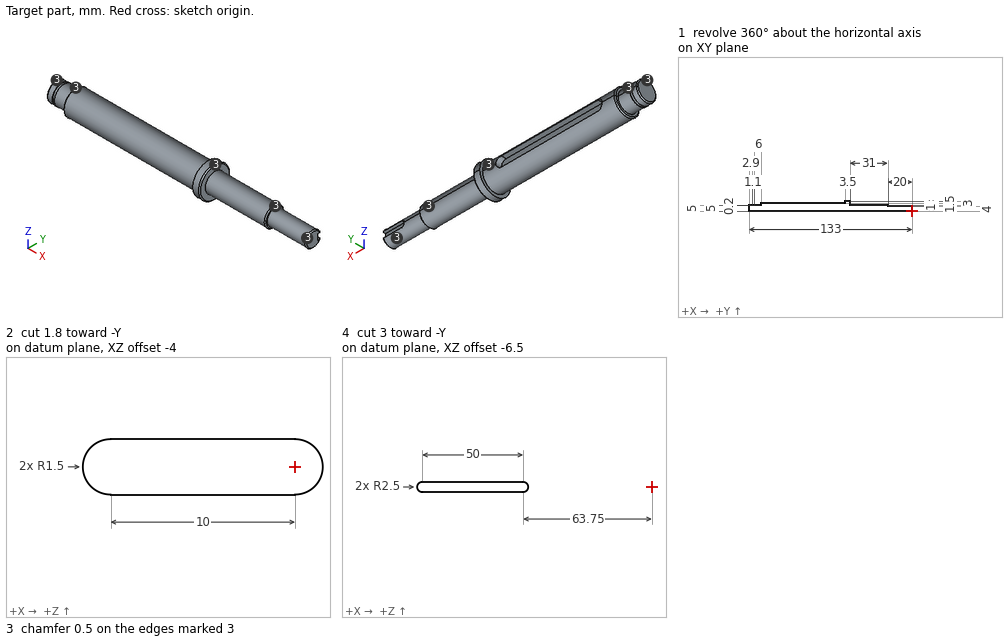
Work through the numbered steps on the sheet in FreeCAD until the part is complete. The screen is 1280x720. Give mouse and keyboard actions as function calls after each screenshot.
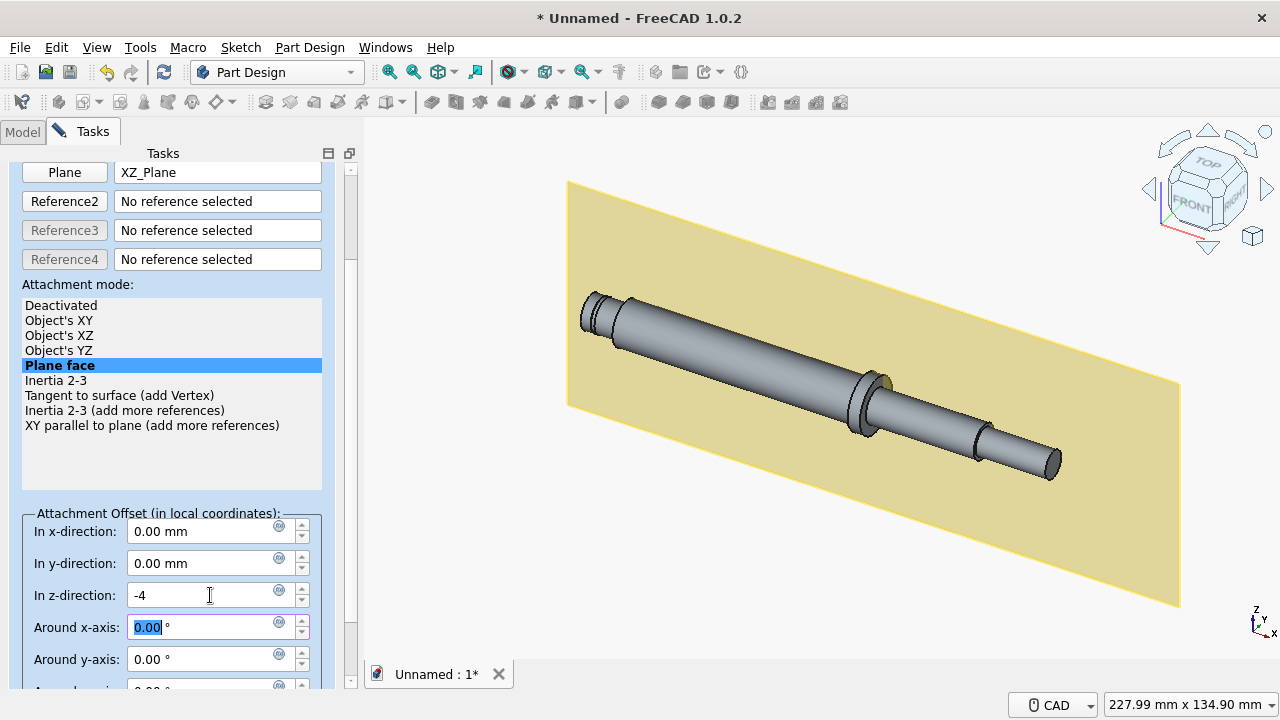
scroll(351, 426, up, 3)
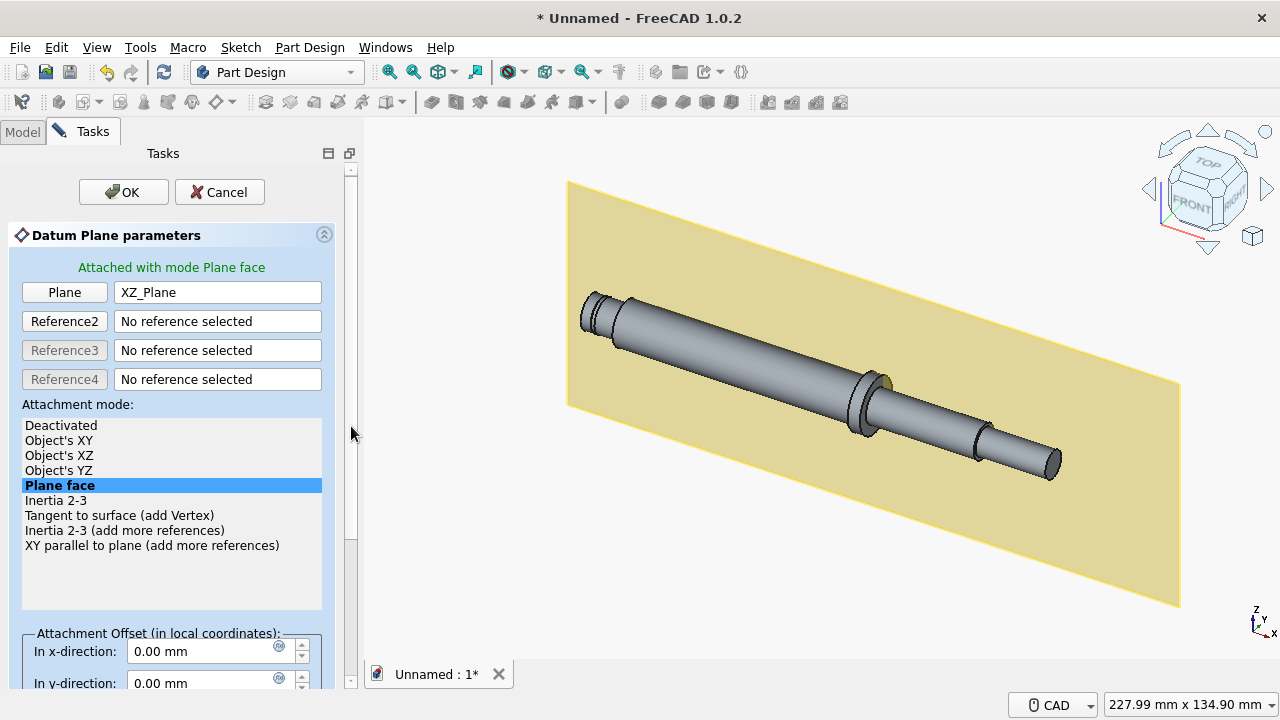
click(124, 192)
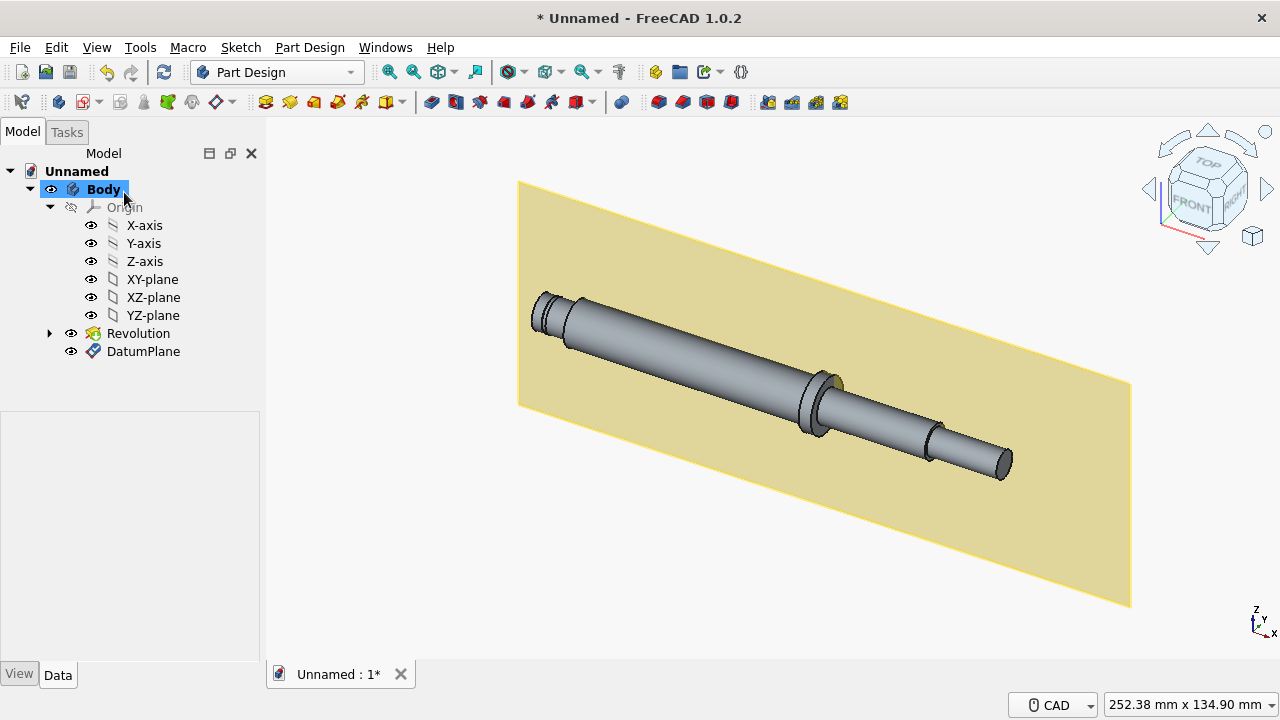
click(116, 351)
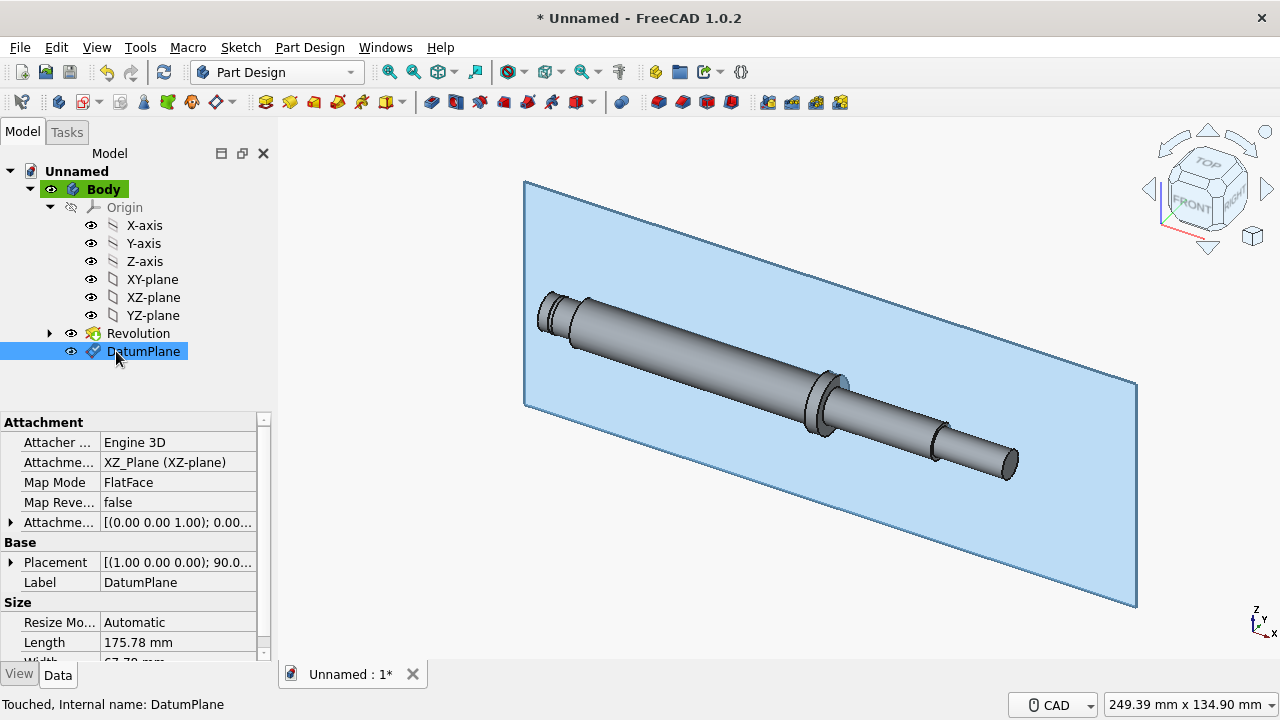
click(84, 102)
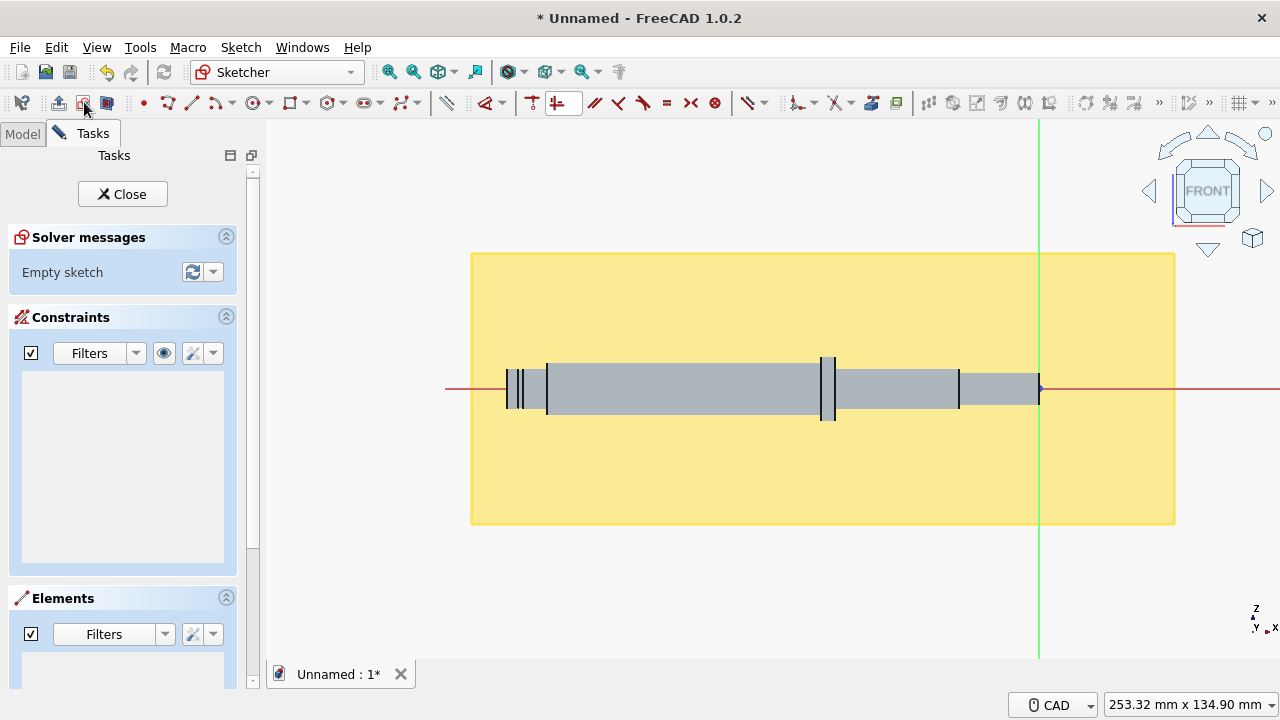
key(q)
key(s)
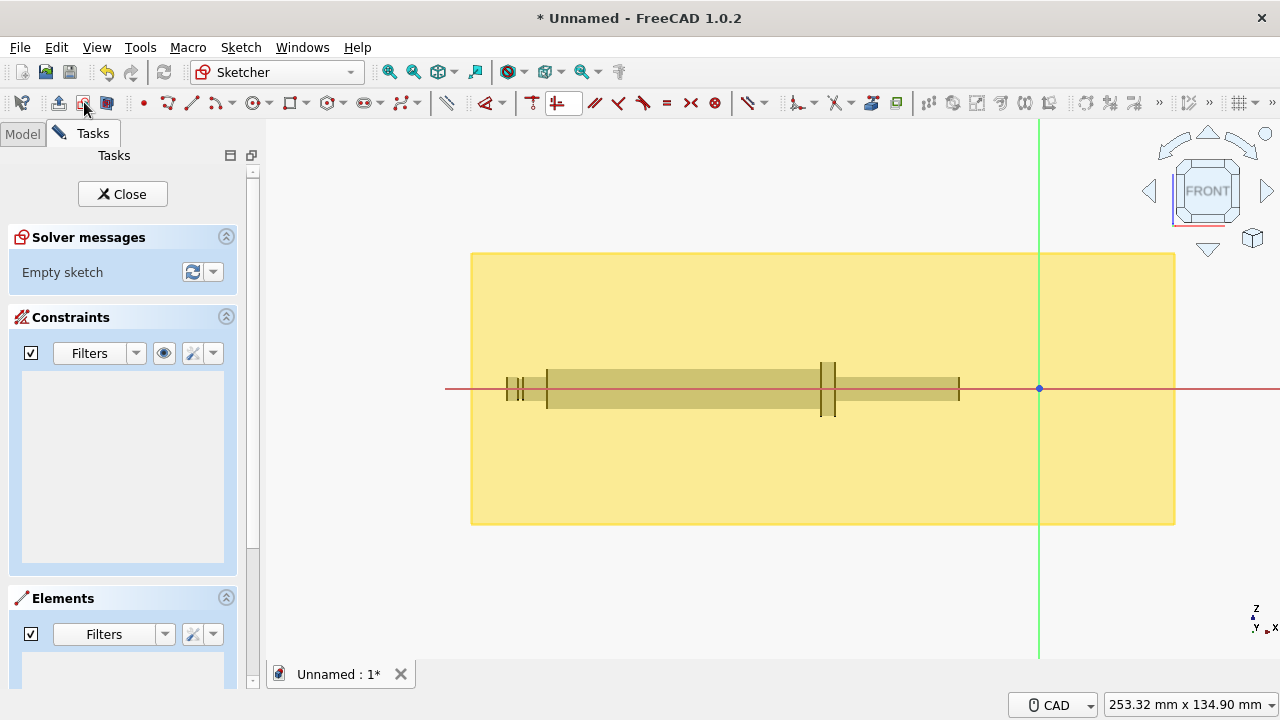
scroll(1051, 389, up, 12)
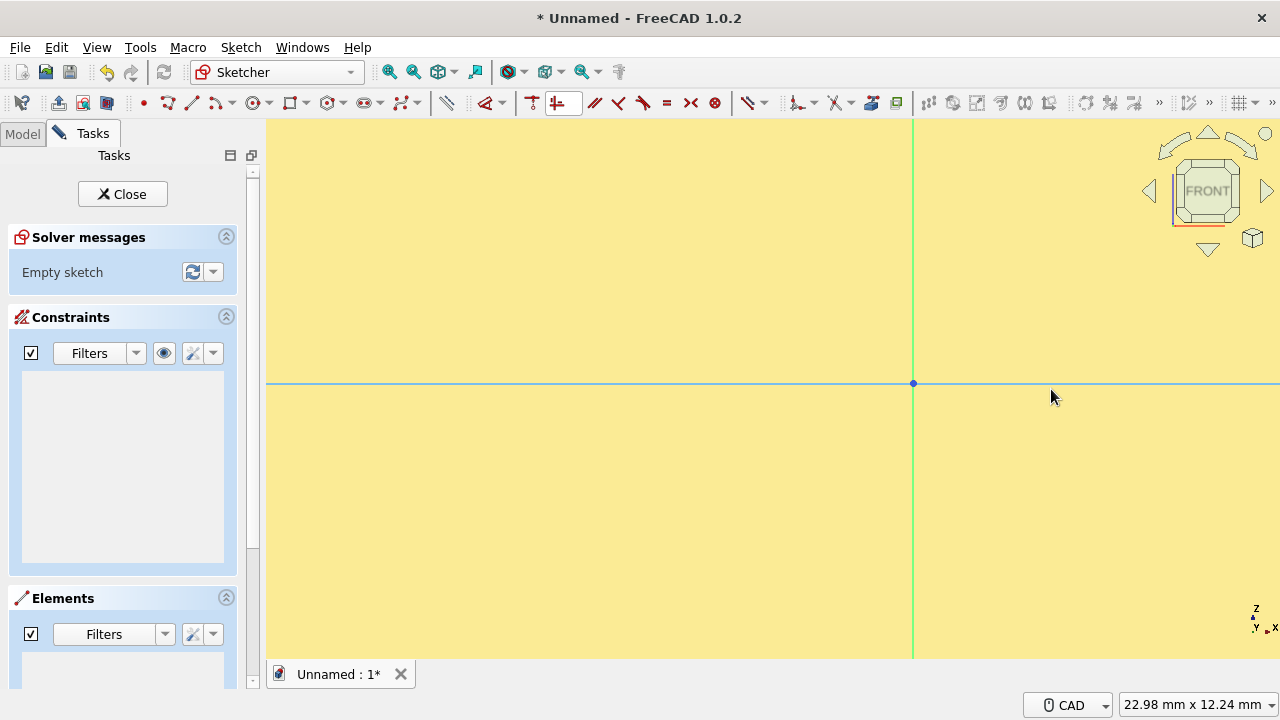
key(g)
key(s)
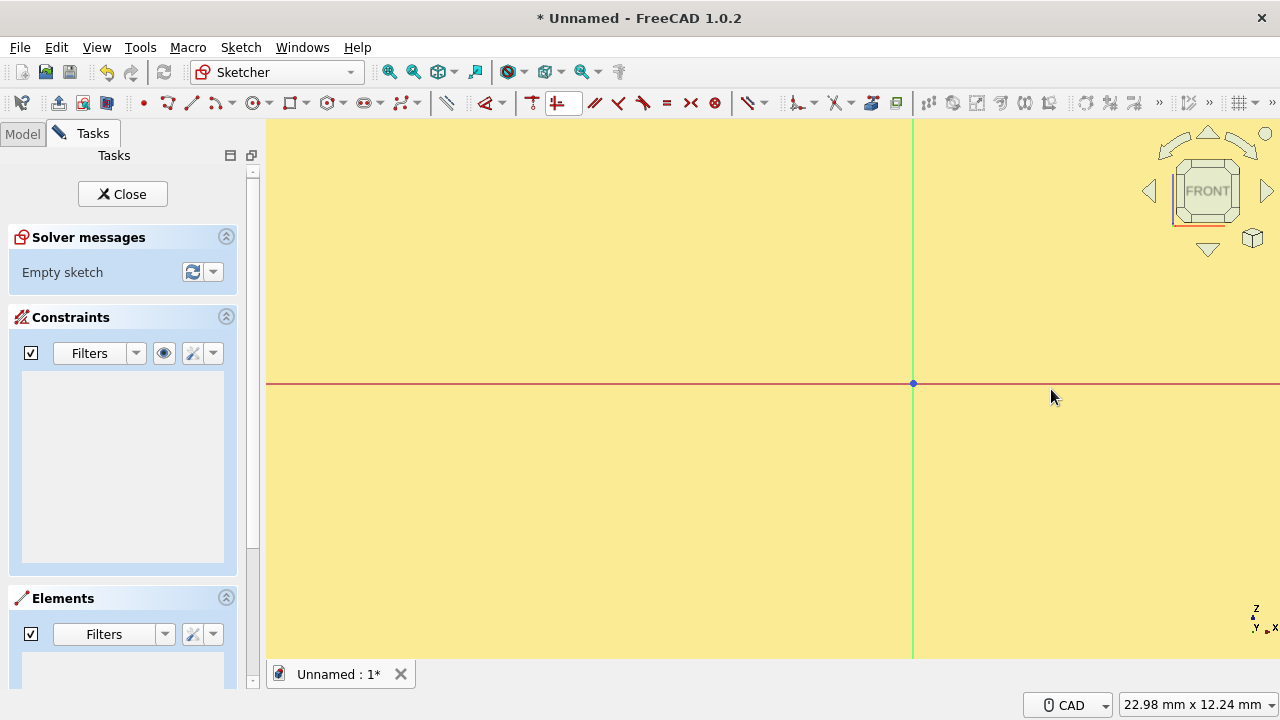
click(913, 384)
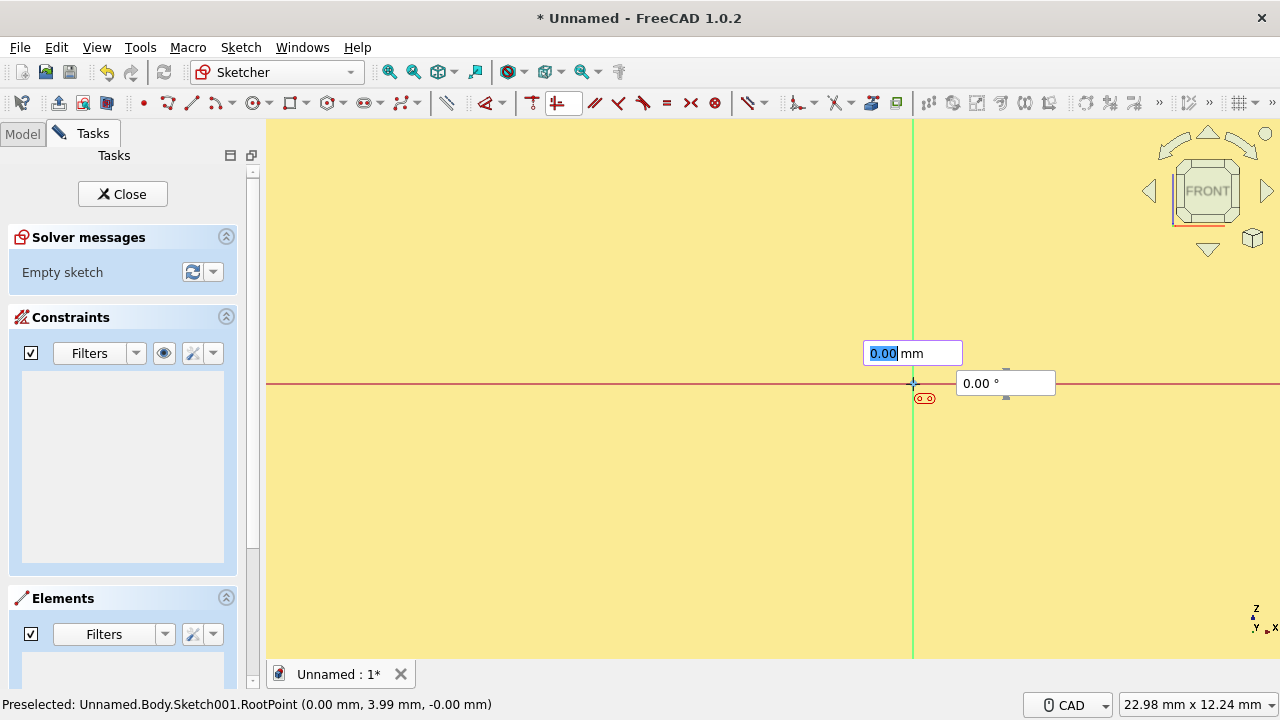
click(472, 375)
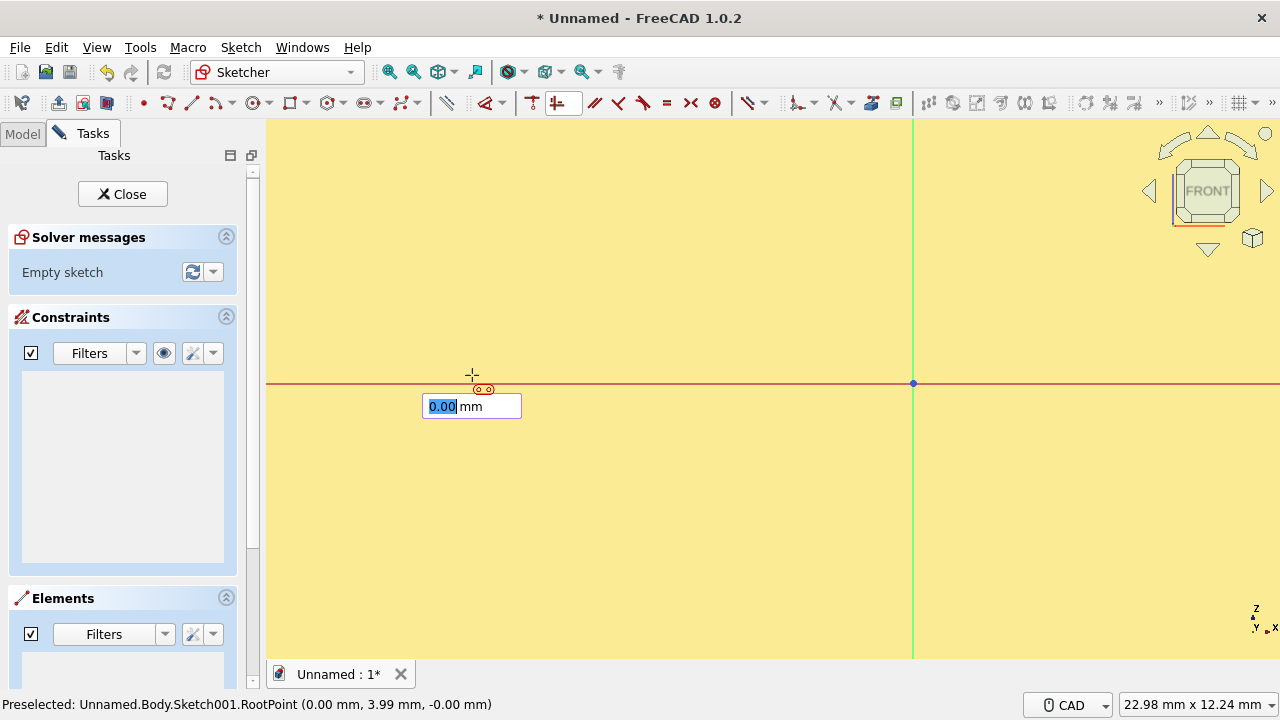
click(692, 450)
key(Escape)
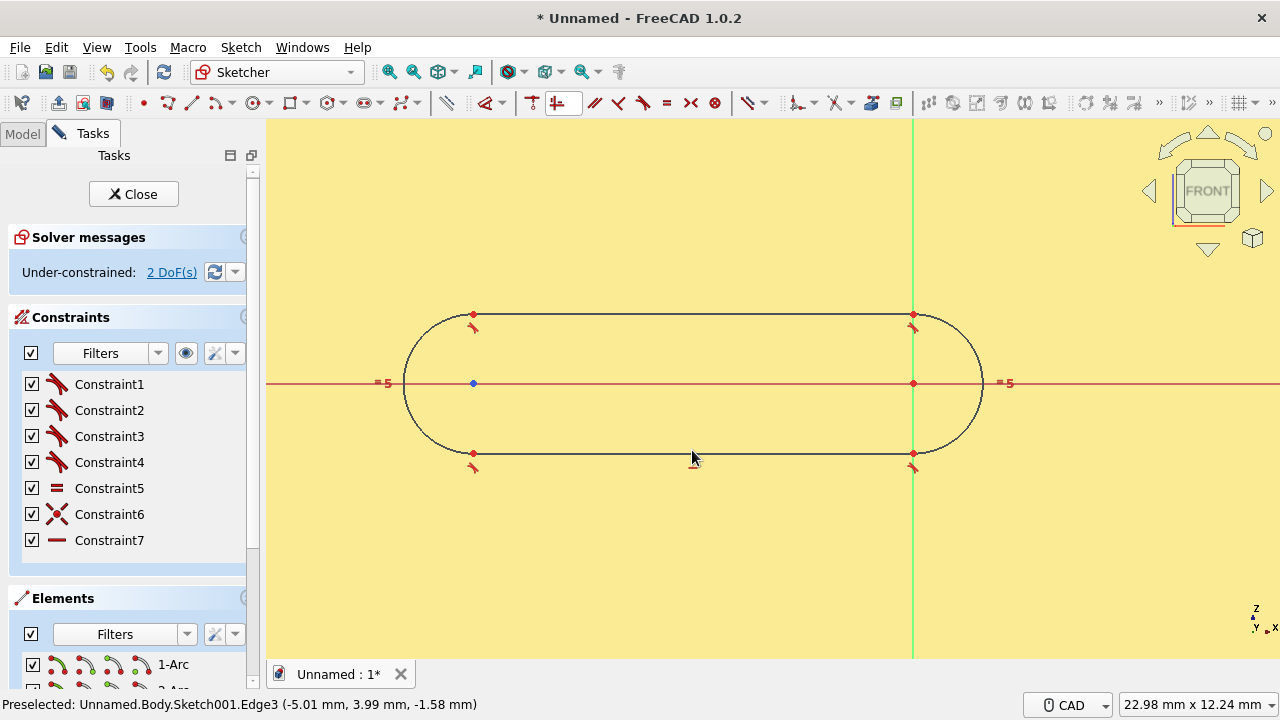
click(486, 104)